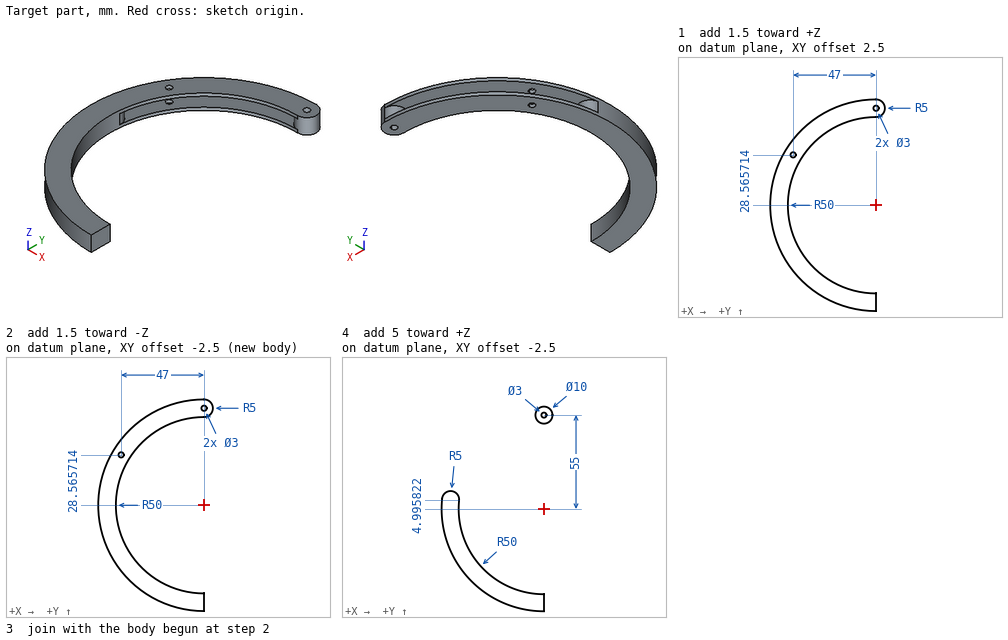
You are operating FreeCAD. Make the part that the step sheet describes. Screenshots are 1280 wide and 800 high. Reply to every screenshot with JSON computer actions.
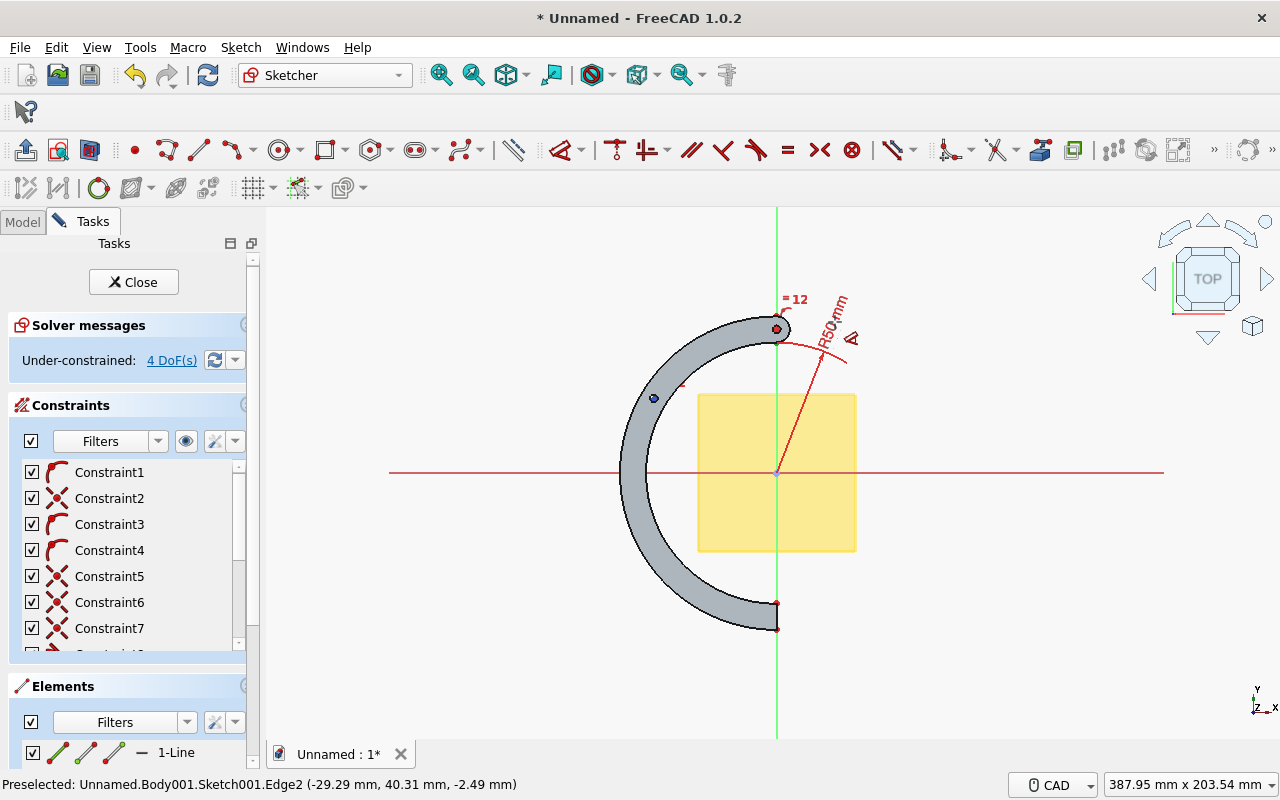
{"action": "scroll", "coordinate": [787, 337], "scroll_direction": "up", "scroll_amount": 6}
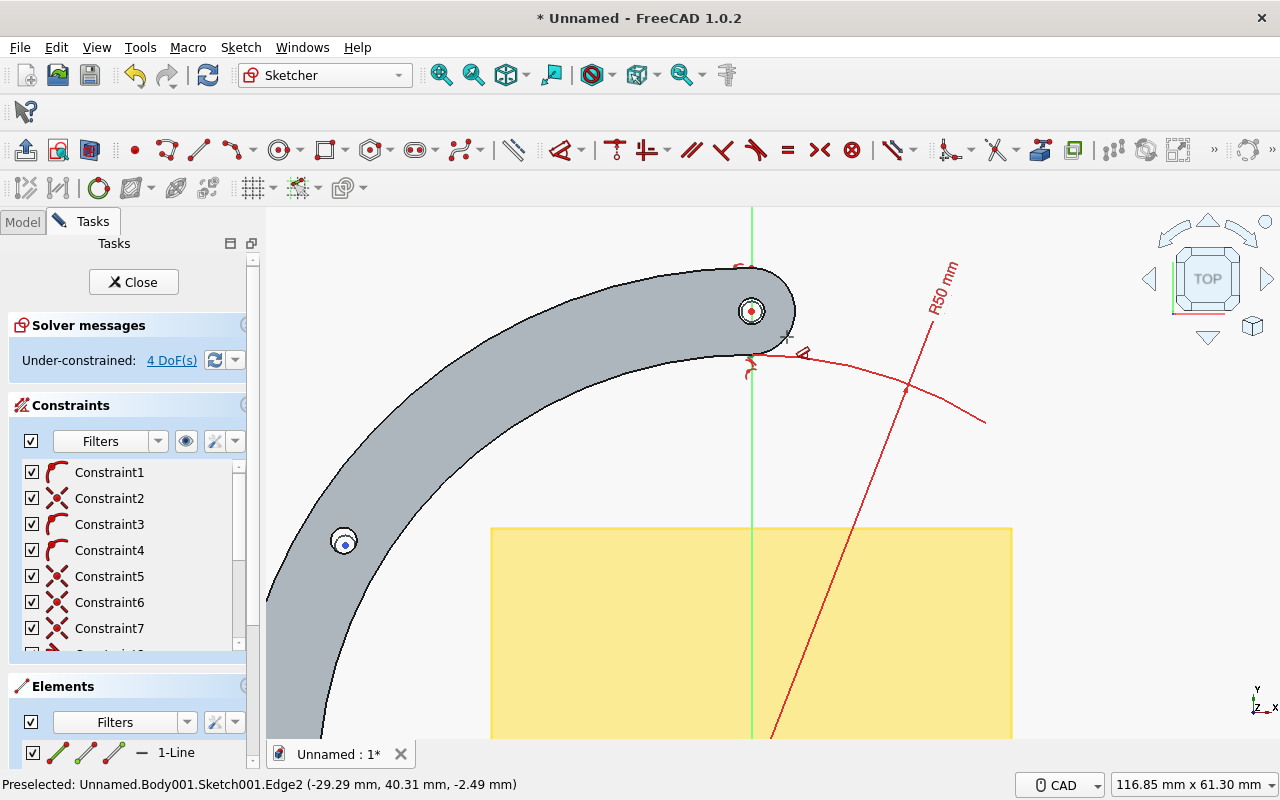
{"action": "left_click", "coordinate": [786, 337]}
{"action": "left_click", "coordinate": [812, 356]}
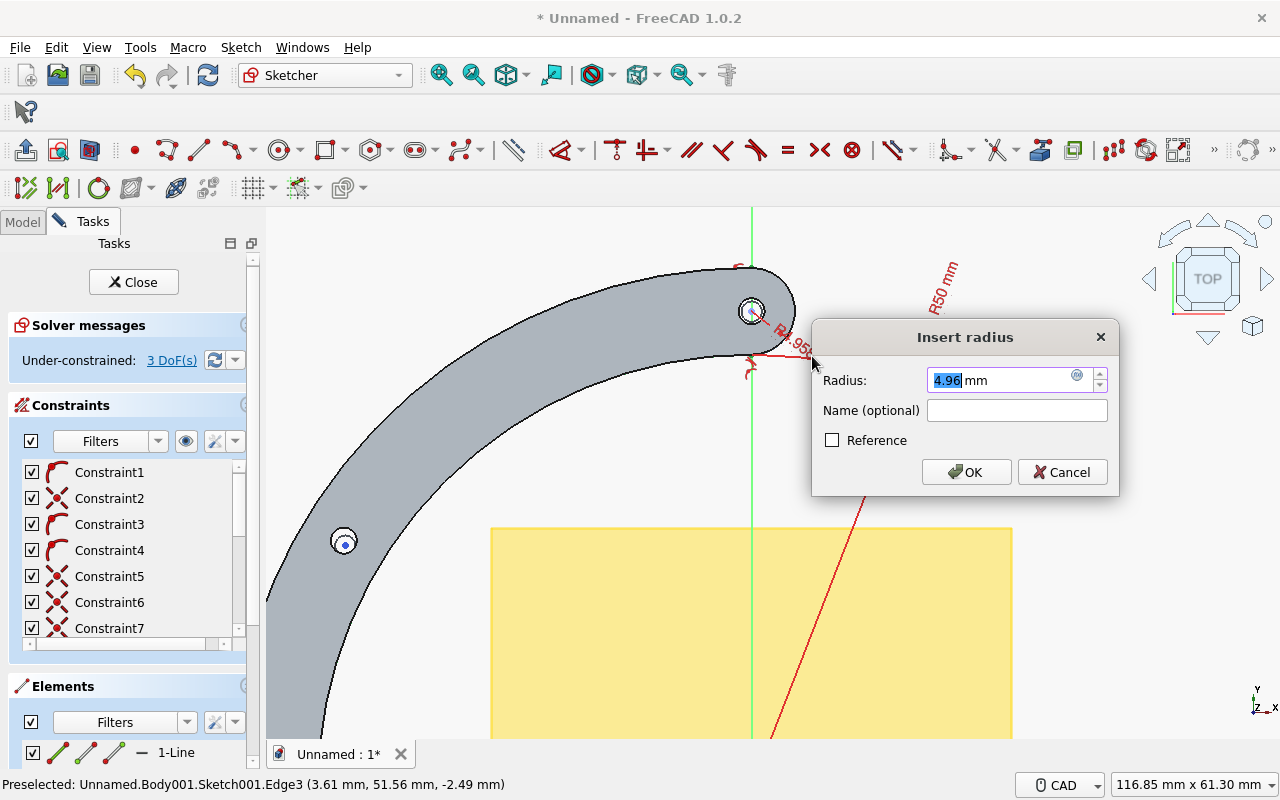
{"action": "type", "text": "5"}
{"action": "key", "text": "Return"}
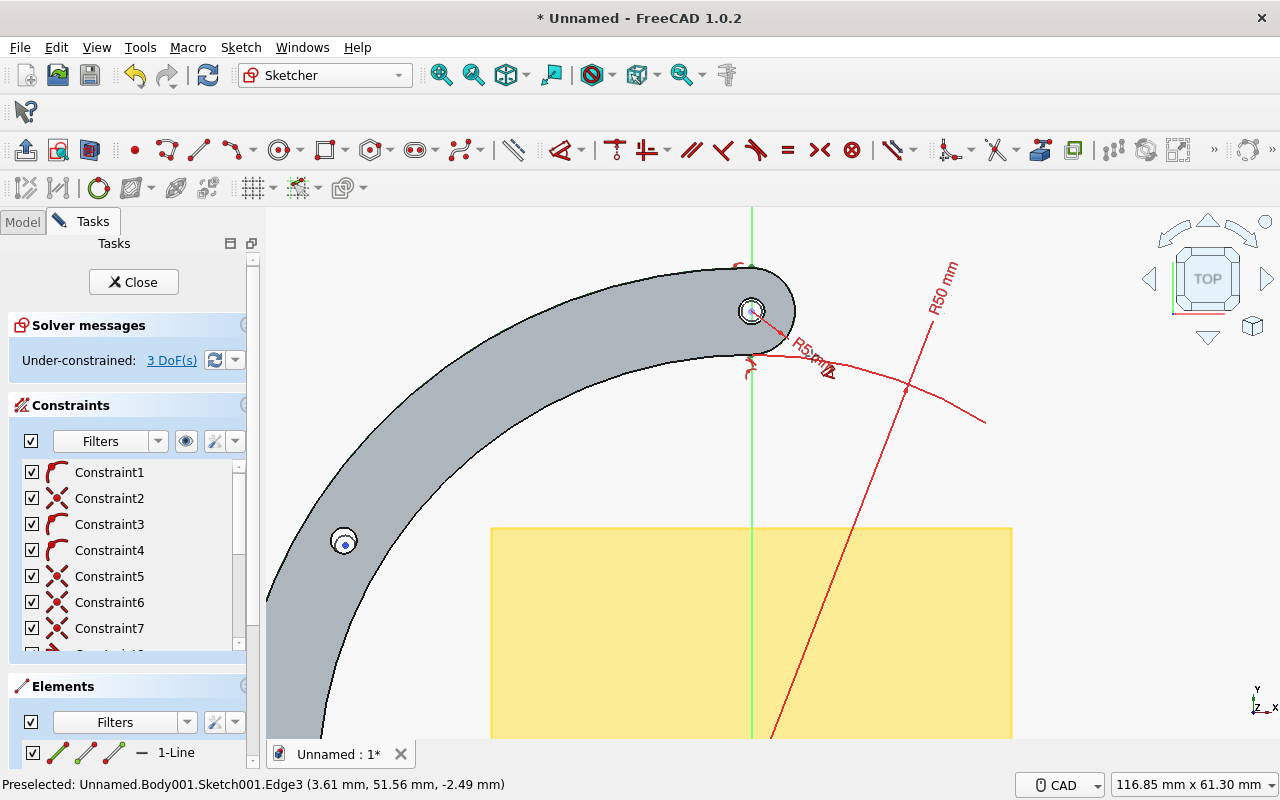
{"action": "scroll", "coordinate": [352, 538], "scroll_direction": "up", "scroll_amount": 3}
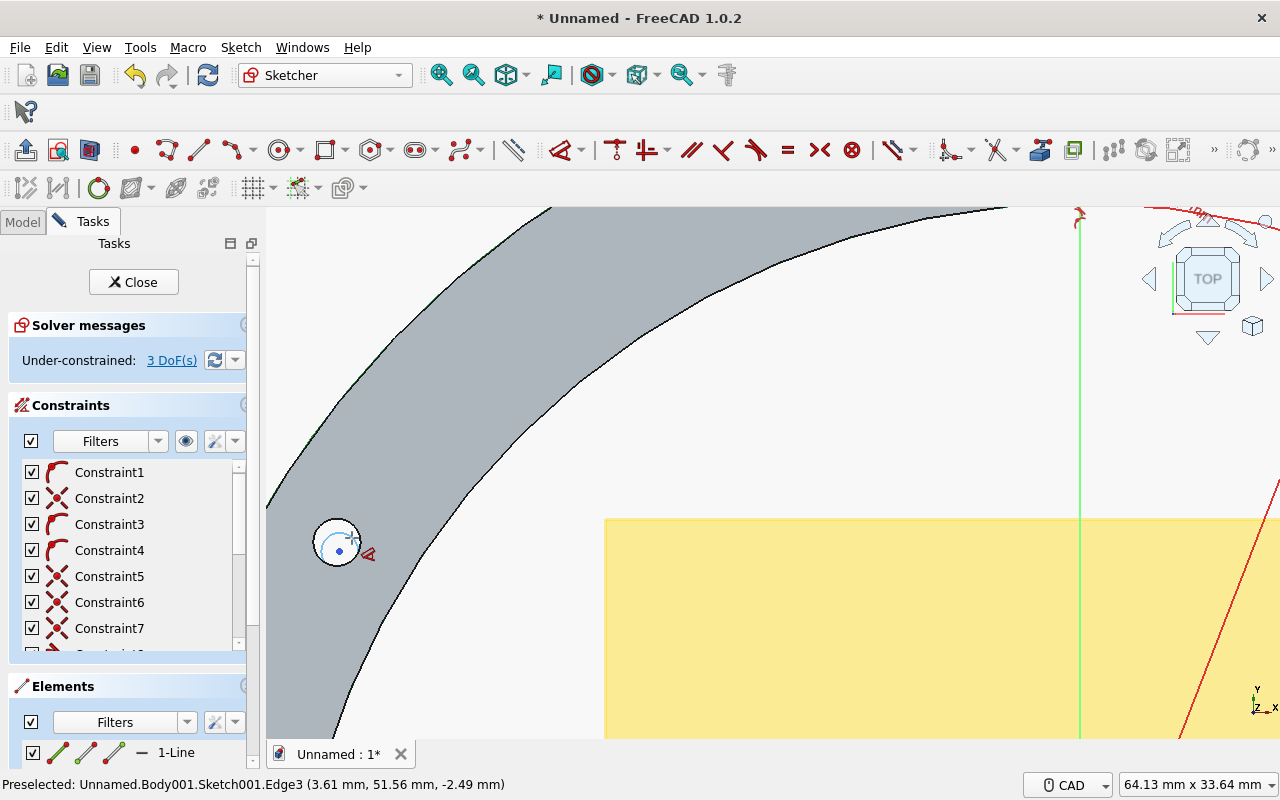
{"action": "left_click", "coordinate": [353, 538]}
{"action": "left_click", "coordinate": [375, 515]}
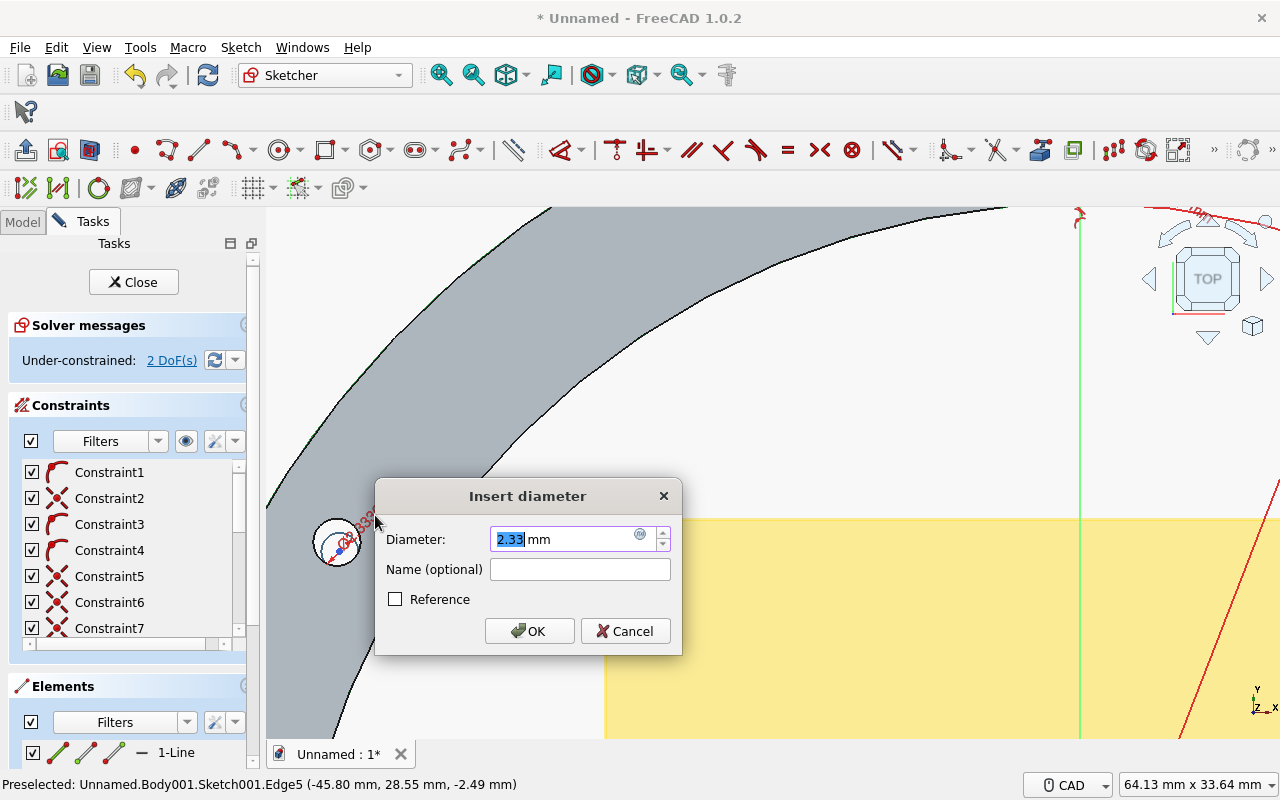
{"action": "type", "text": "3"}
{"action": "key", "text": "Return"}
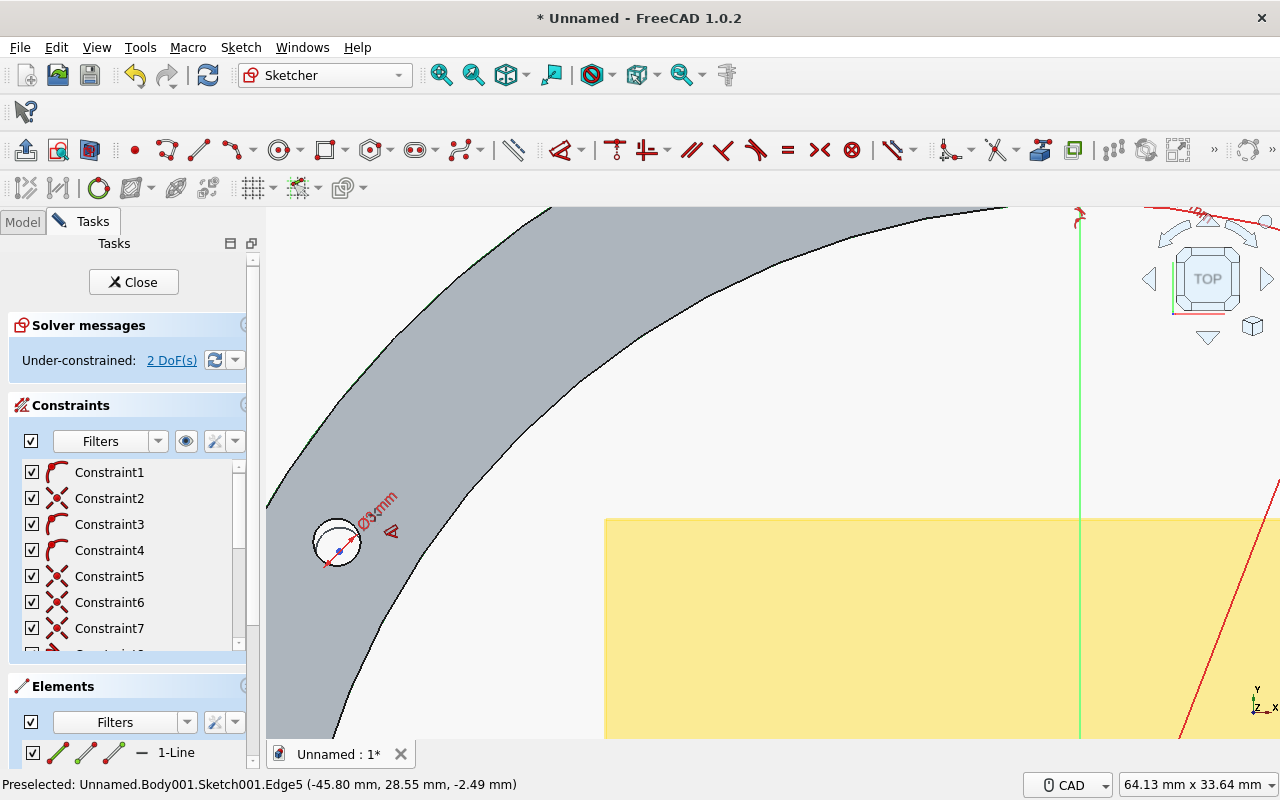
{"action": "scroll", "coordinate": [716, 370], "scroll_direction": "down", "scroll_amount": 9}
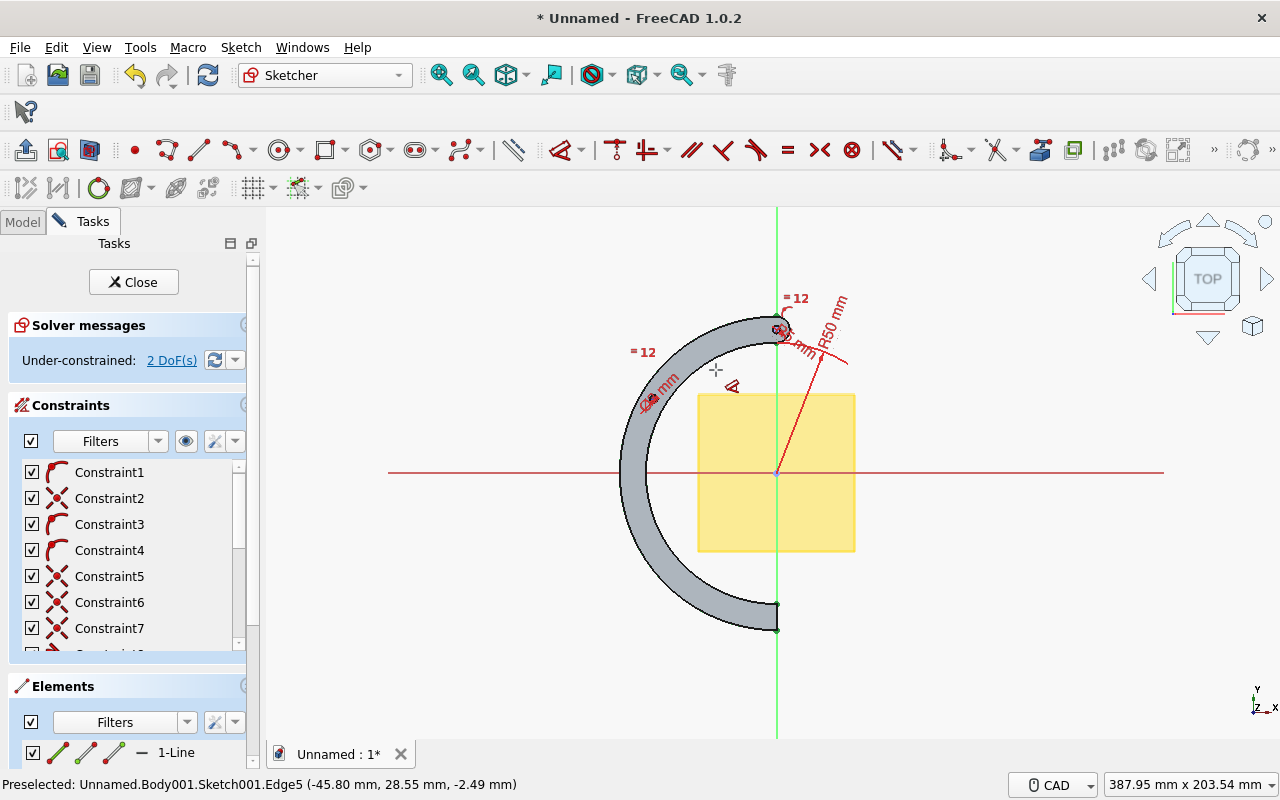
{"action": "left_click", "coordinate": [654, 400]}
{"action": "left_click", "coordinate": [744, 366]}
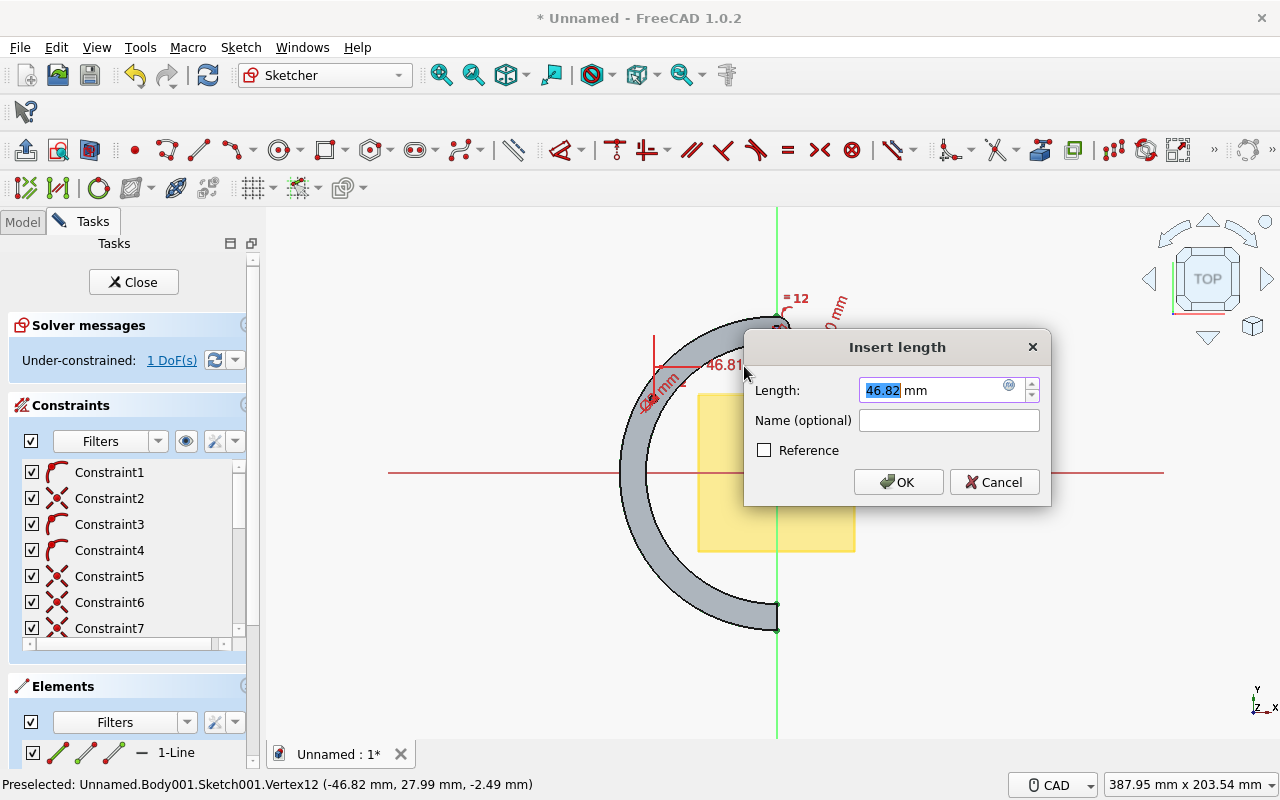
{"action": "type", "text": "47"}
{"action": "key", "text": "Return"}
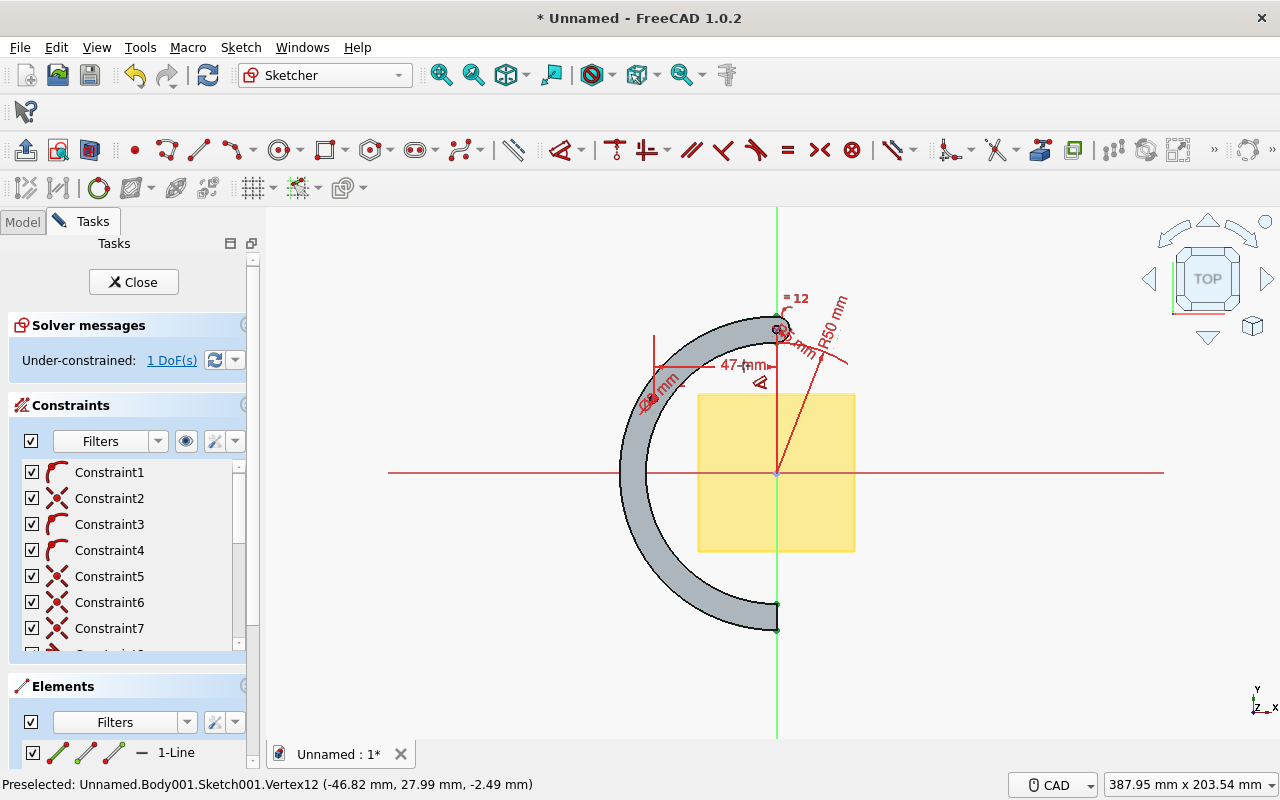
{"action": "left_click", "coordinate": [654, 400]}
{"action": "left_click", "coordinate": [811, 437]}